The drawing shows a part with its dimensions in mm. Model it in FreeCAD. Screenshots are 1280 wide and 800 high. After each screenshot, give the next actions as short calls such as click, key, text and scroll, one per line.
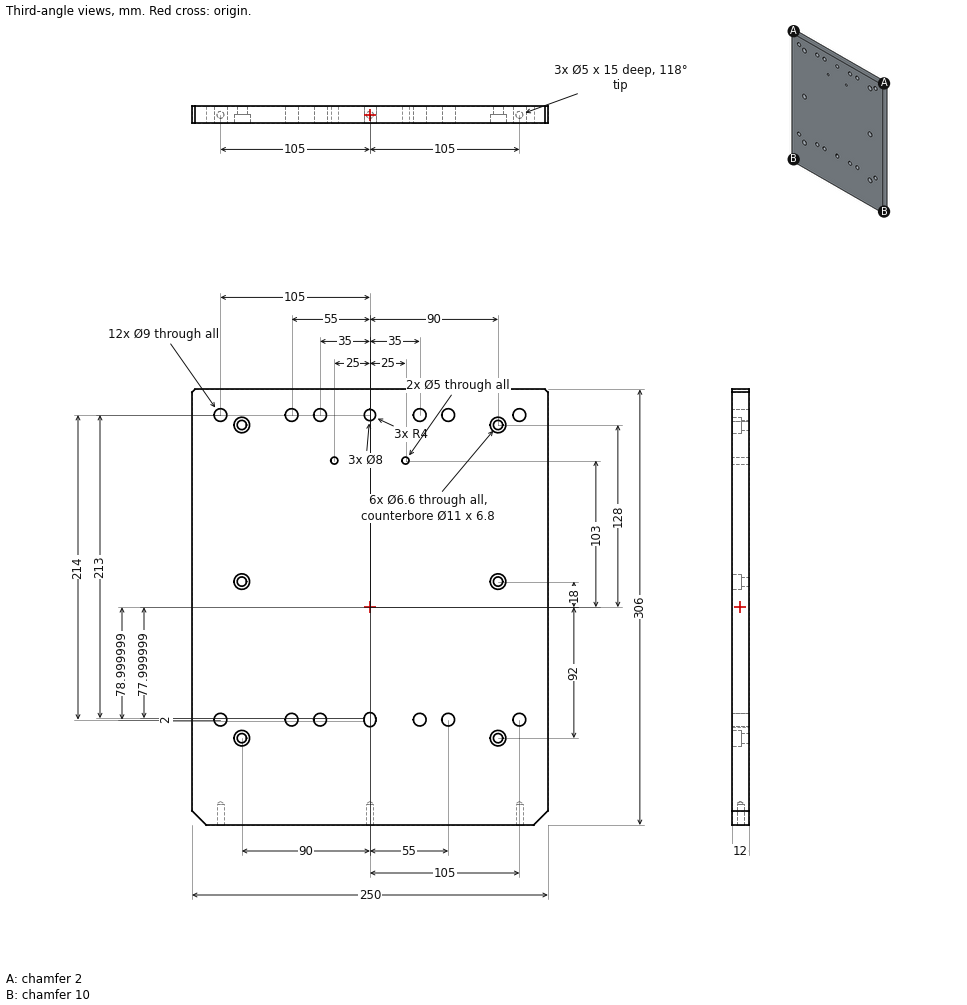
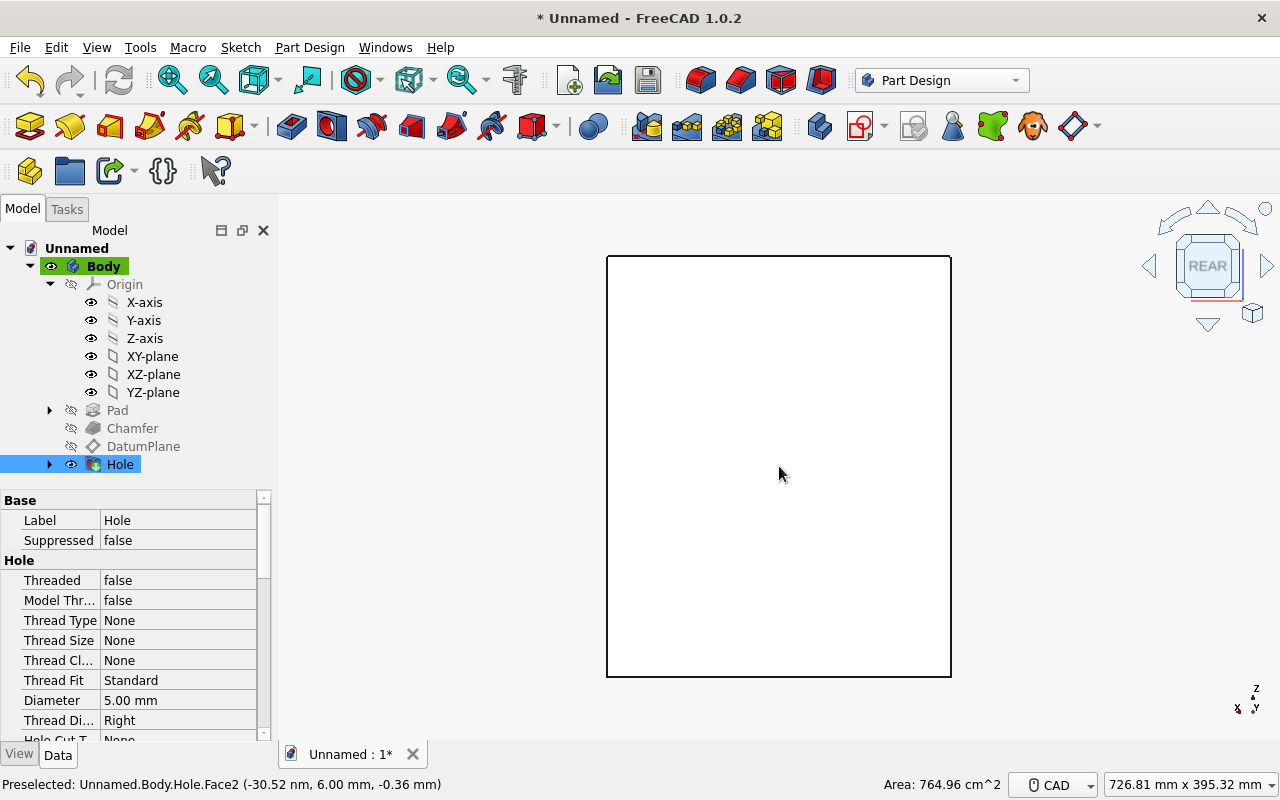
click(860, 126)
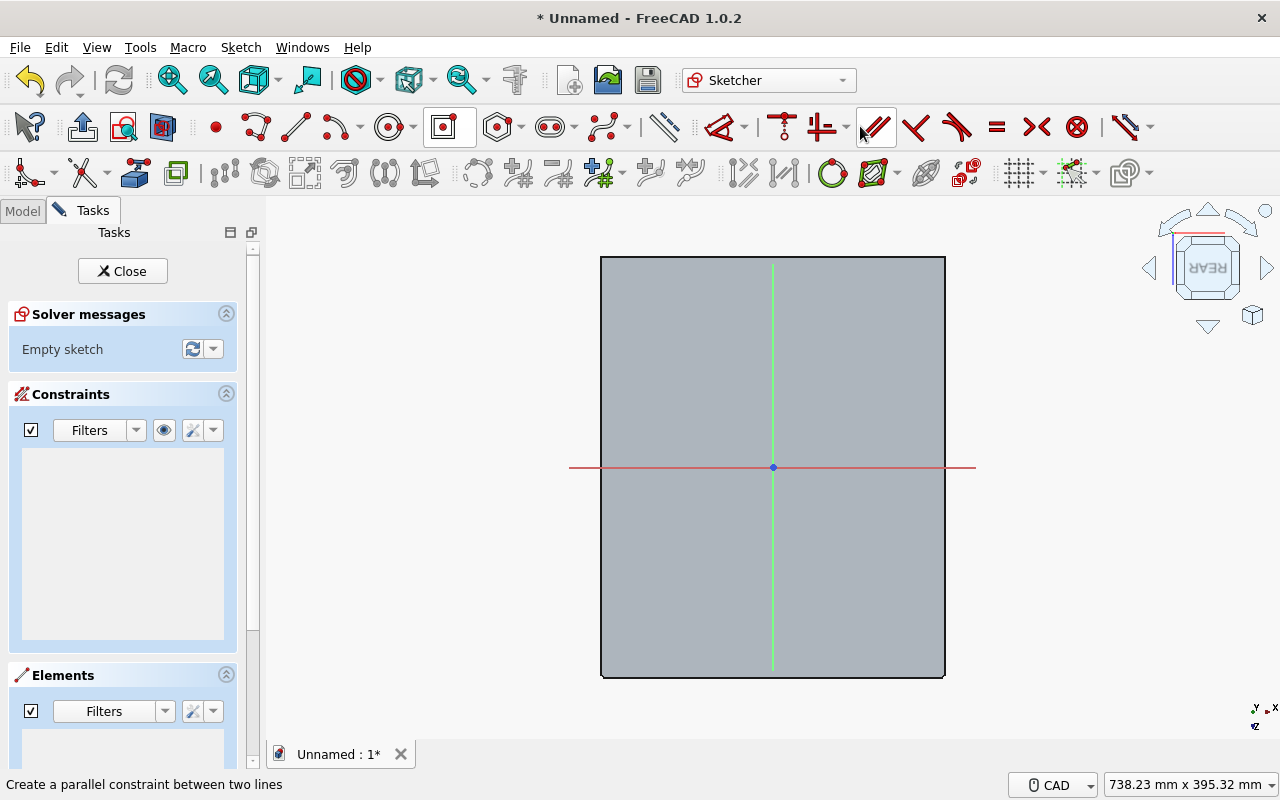
click(390, 128)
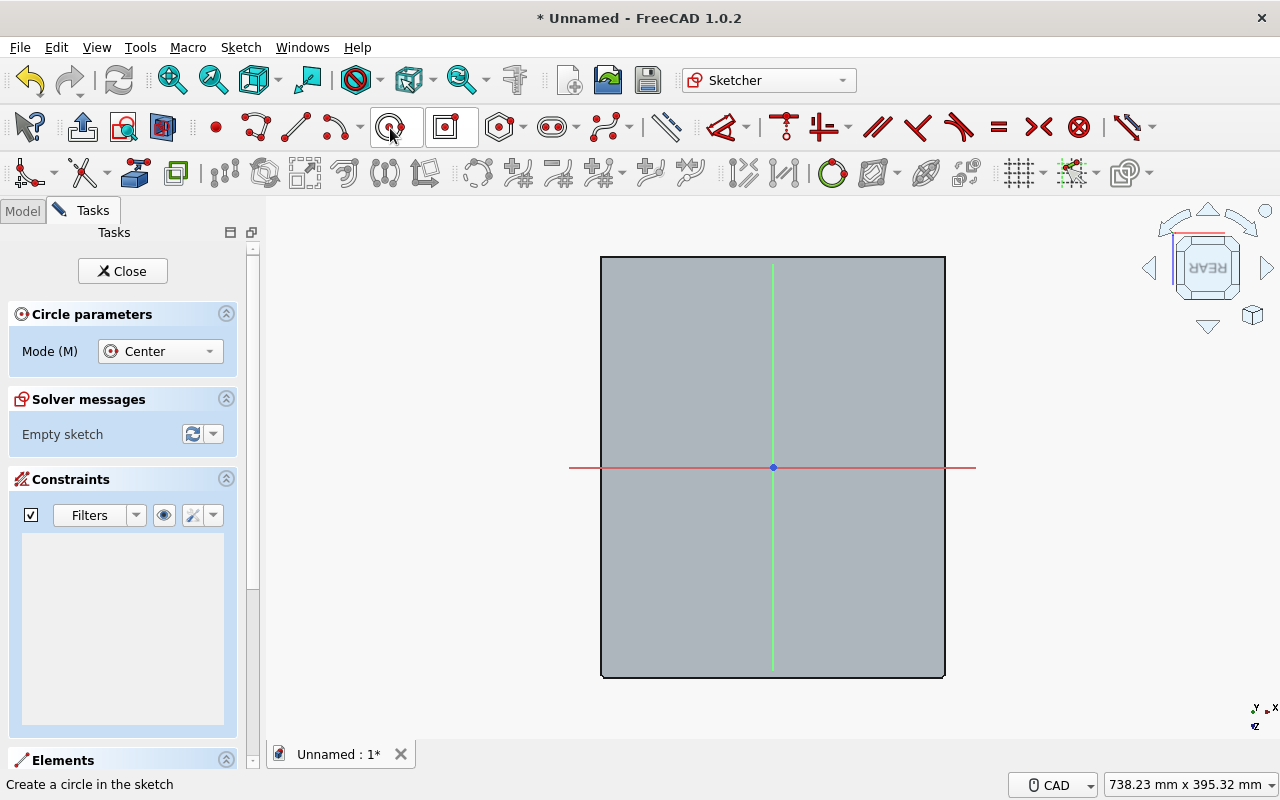
scroll(629, 653, up, 7)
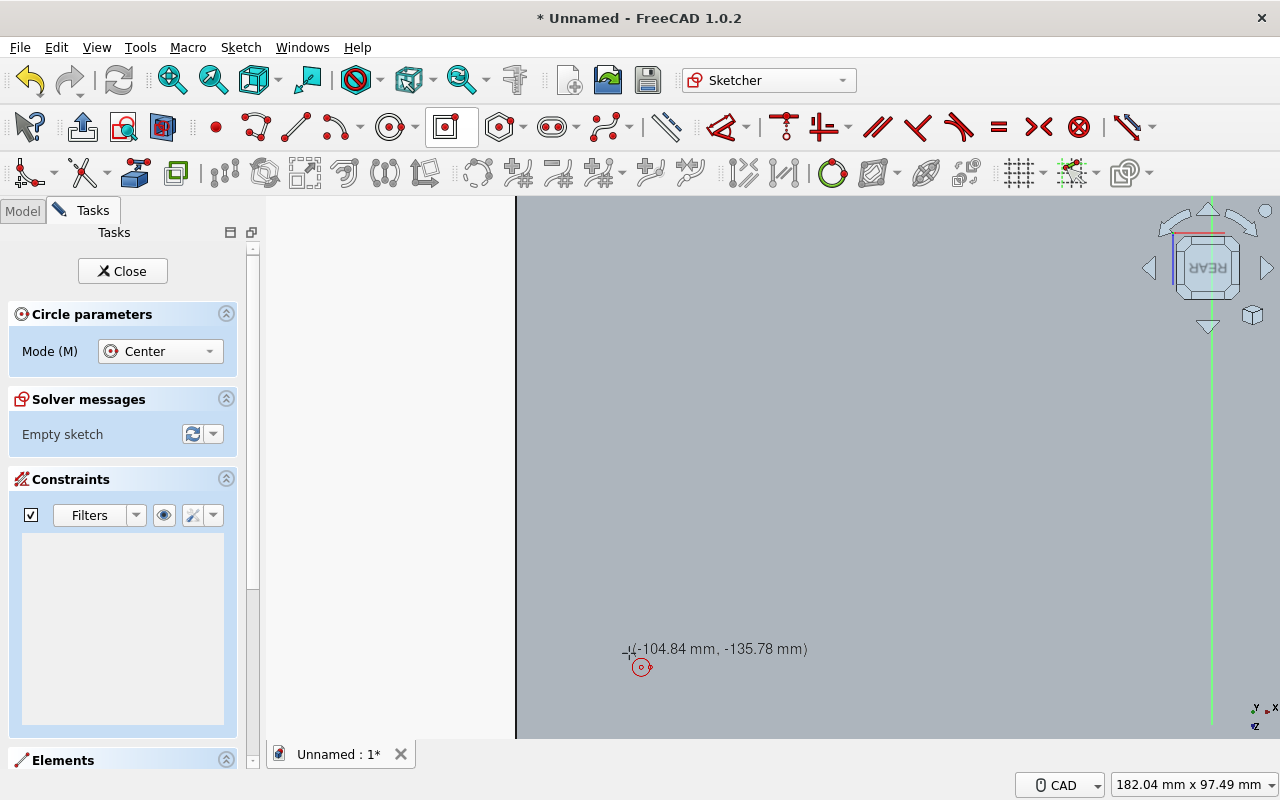
scroll(486, 646, down, 6)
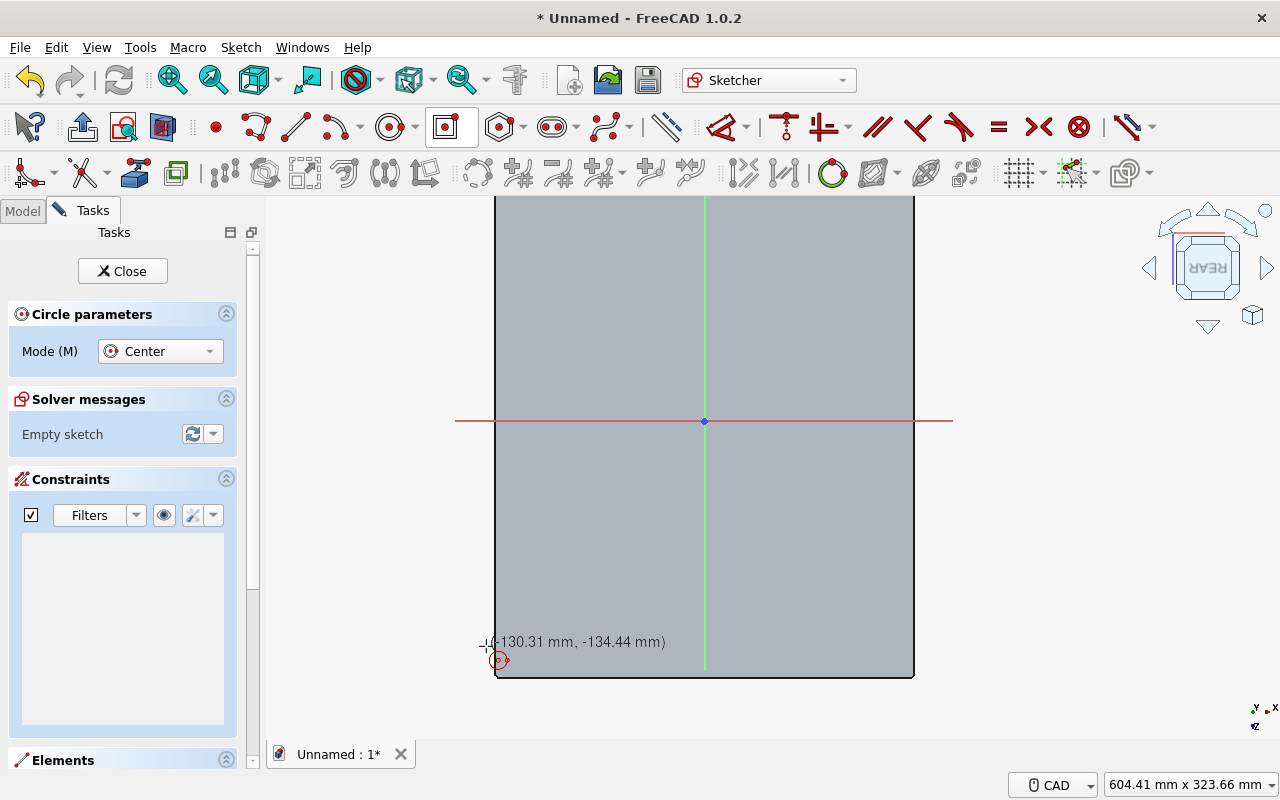
click(529, 648)
move(534, 642)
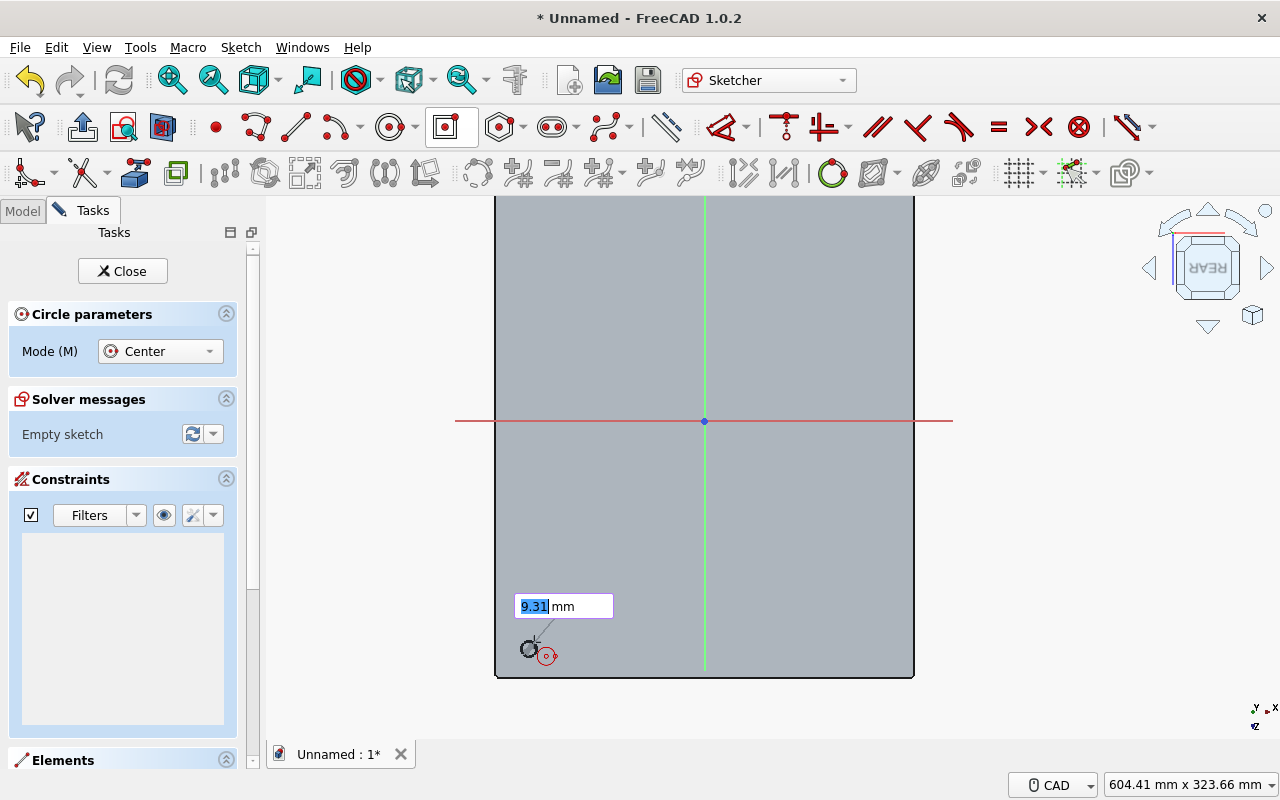
text(9)
key(Return)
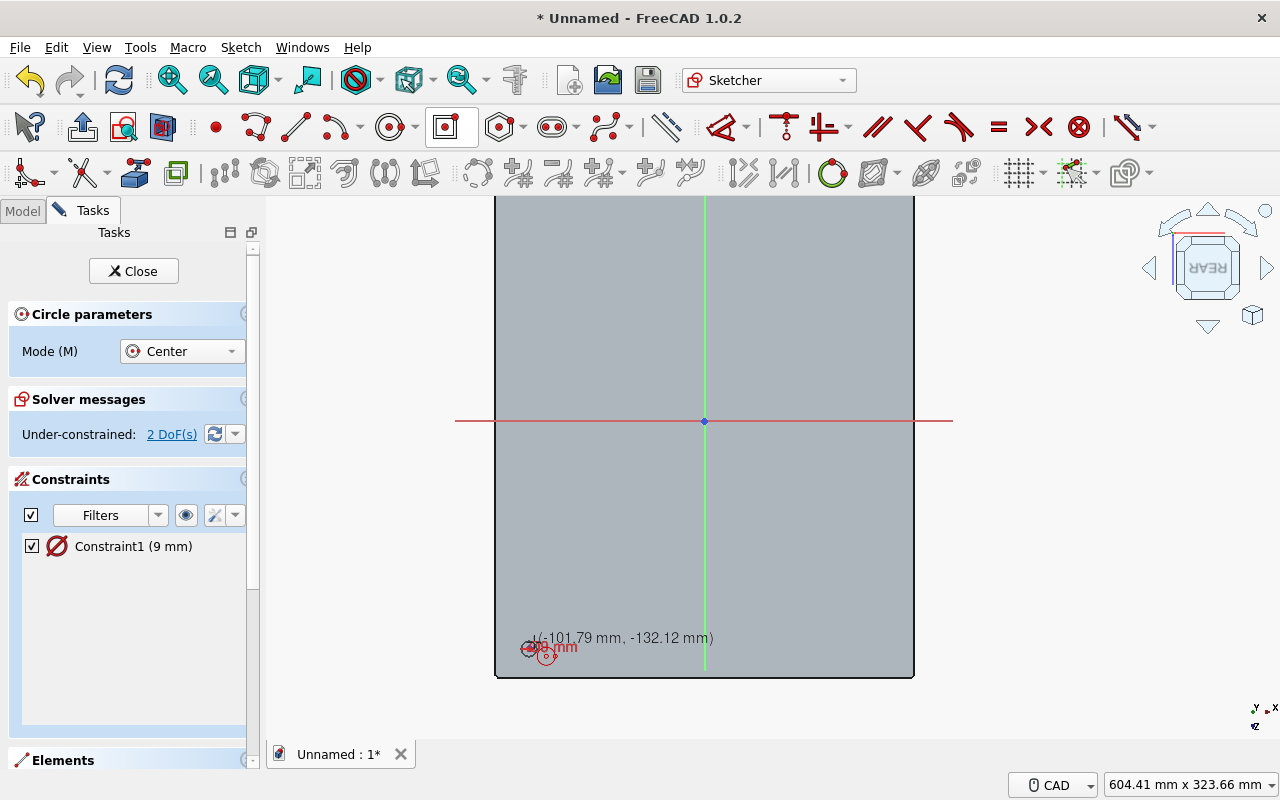
scroll(613, 648, up, 6)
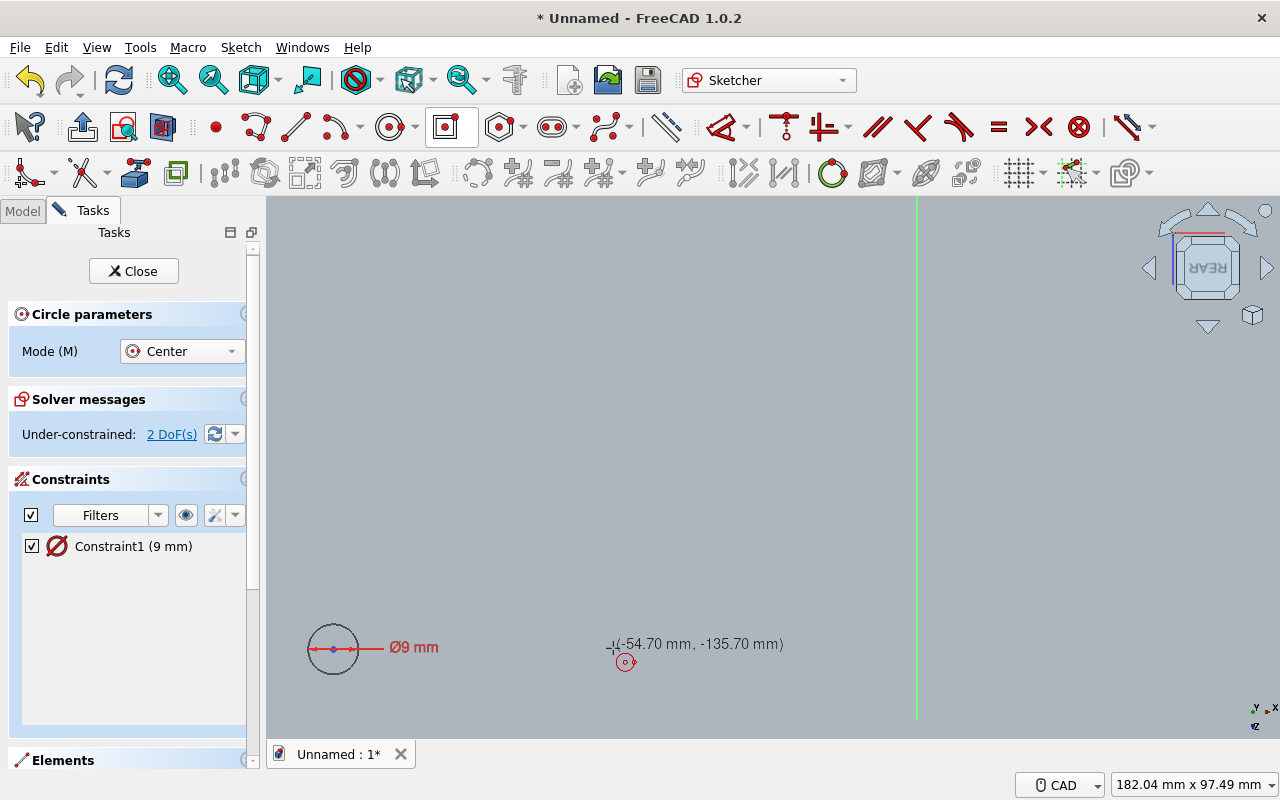
scroll(613, 648, down, 6)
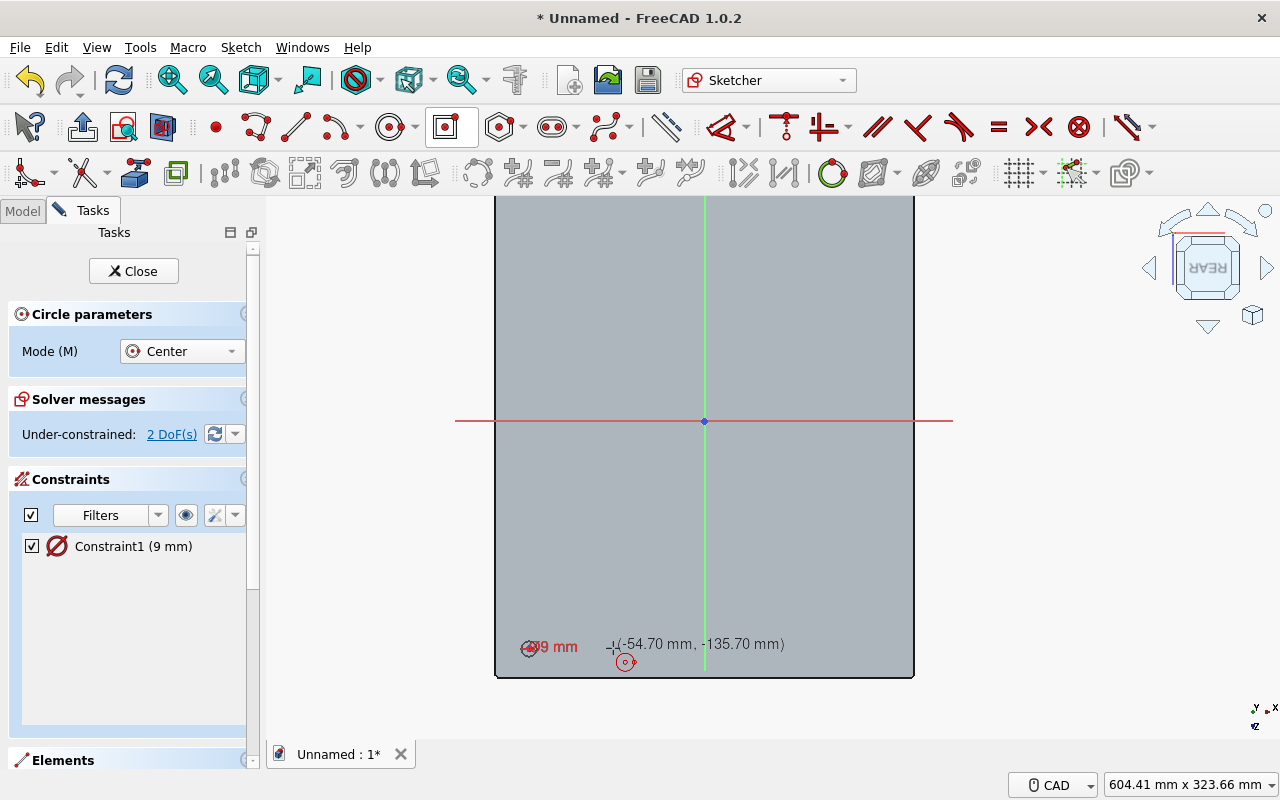
click(613, 648)
move(618, 642)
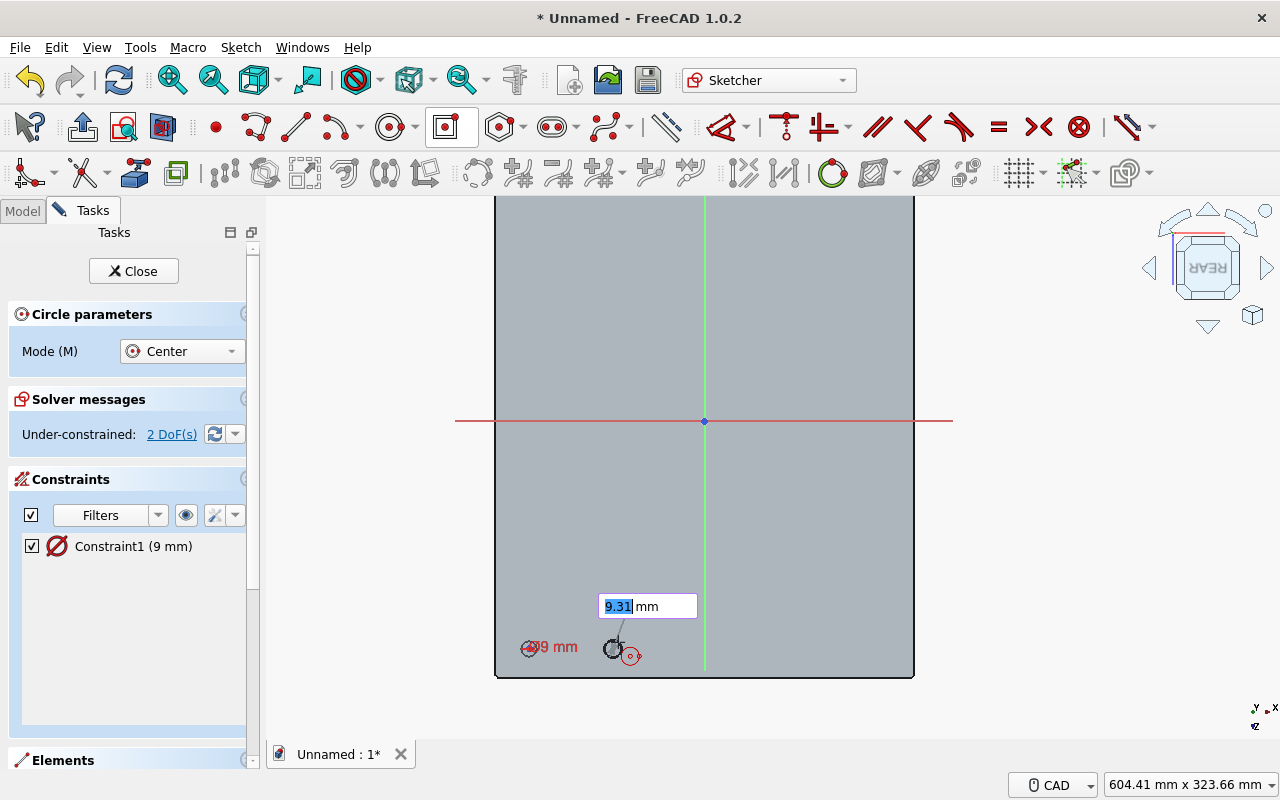
text(9)
key(Return)